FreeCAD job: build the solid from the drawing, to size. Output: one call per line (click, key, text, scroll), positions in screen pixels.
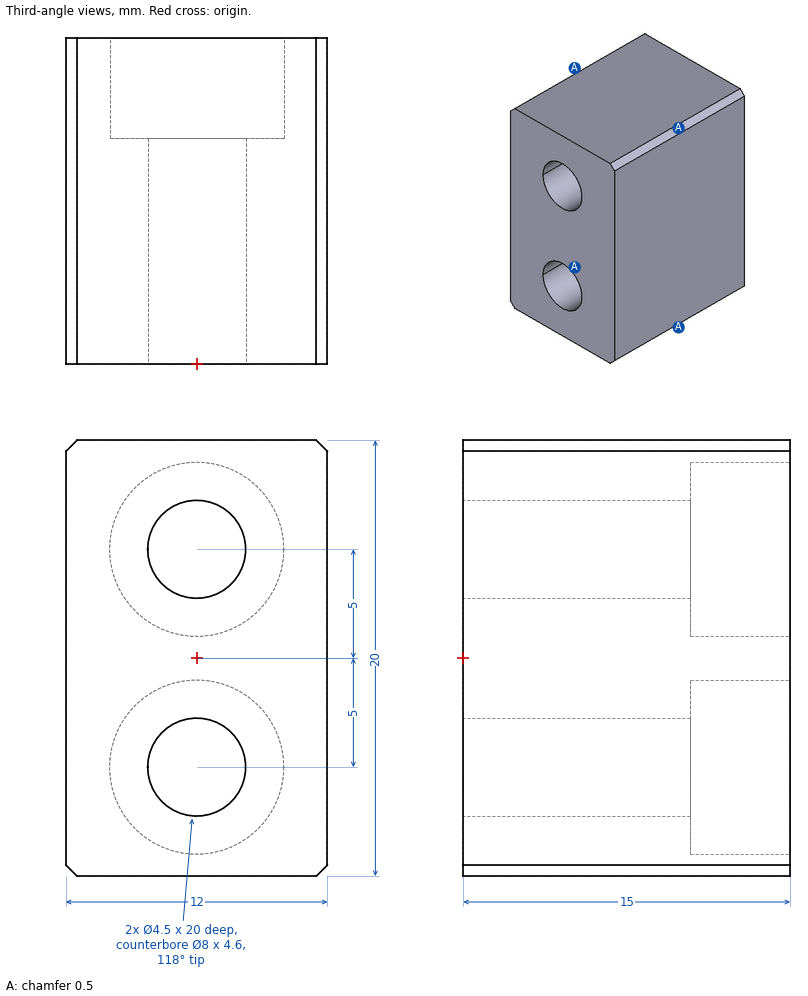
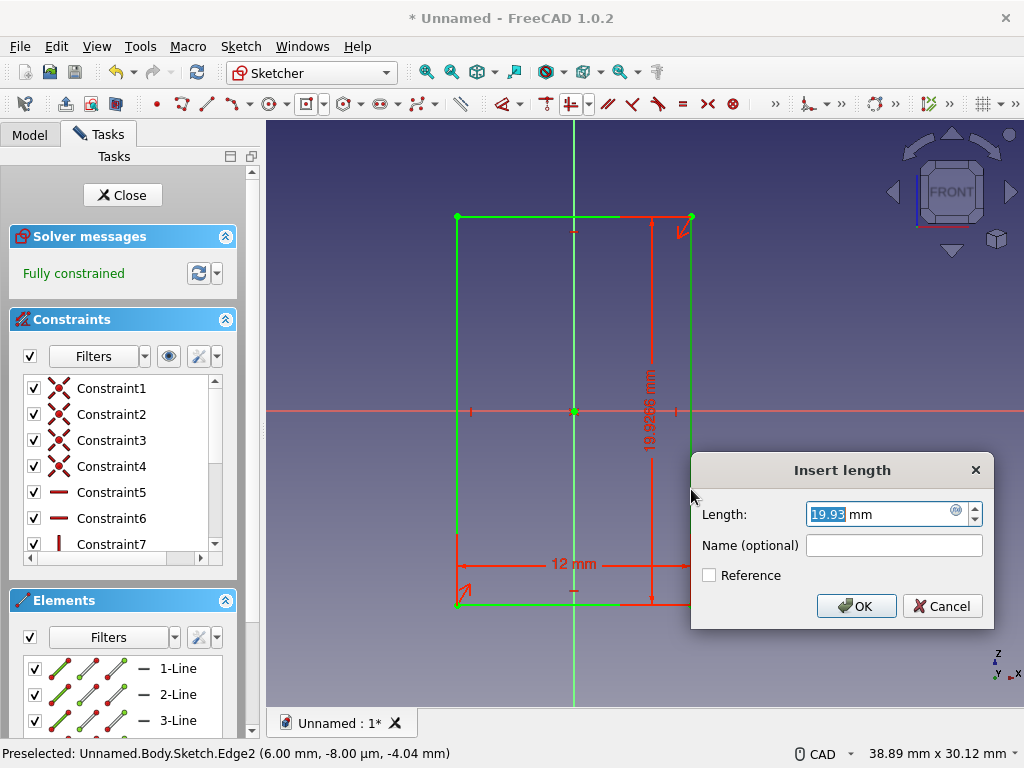
text(20)
key(Return)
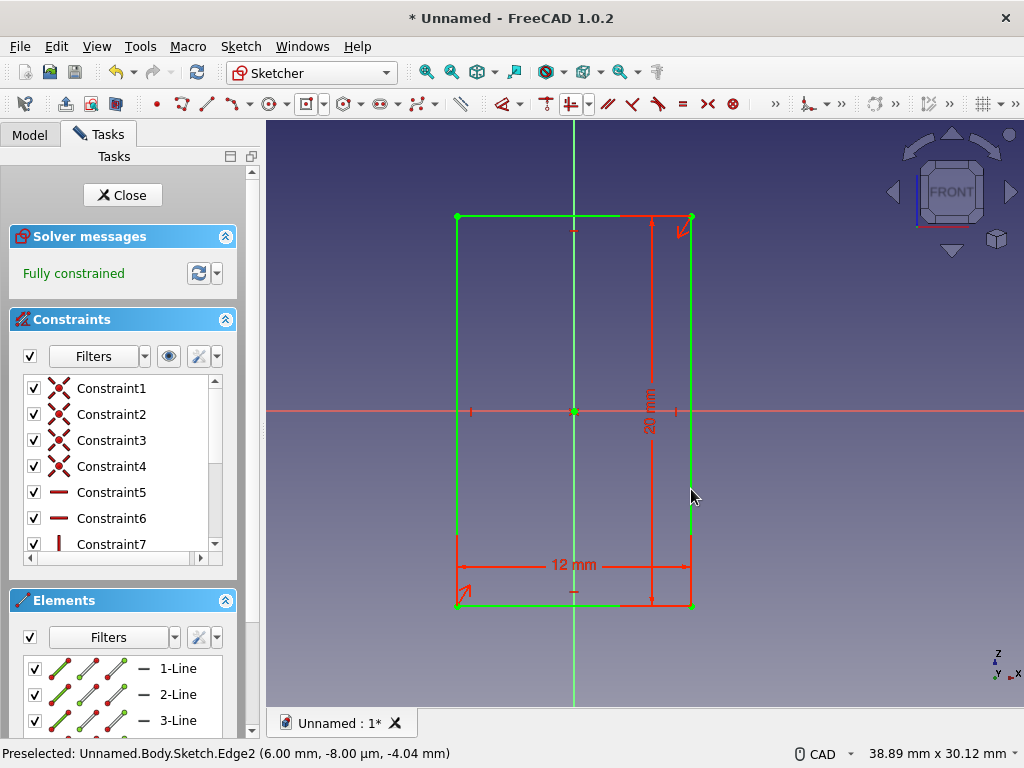
click(123, 195)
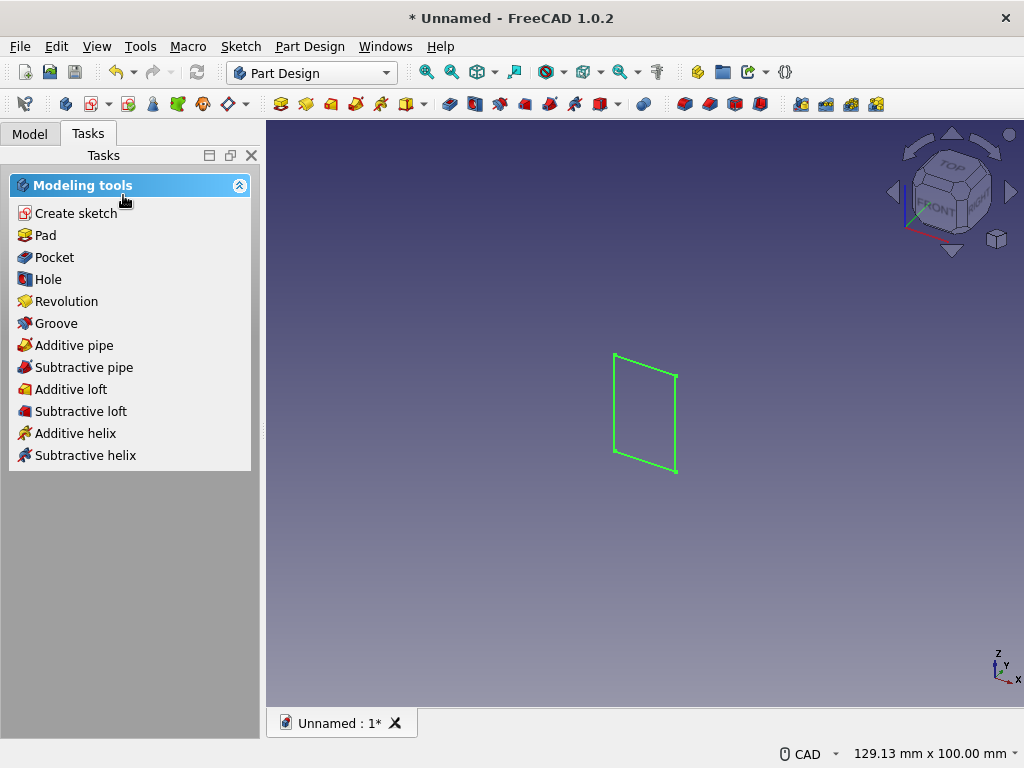
click(281, 104)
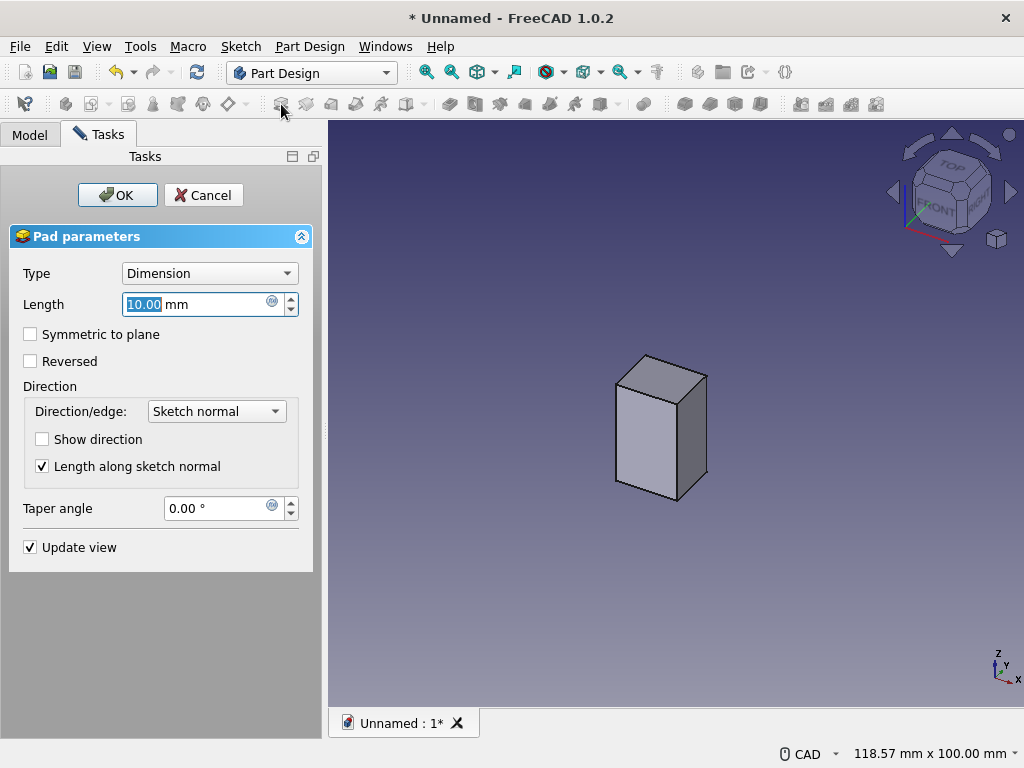
text(15)
key(Tab)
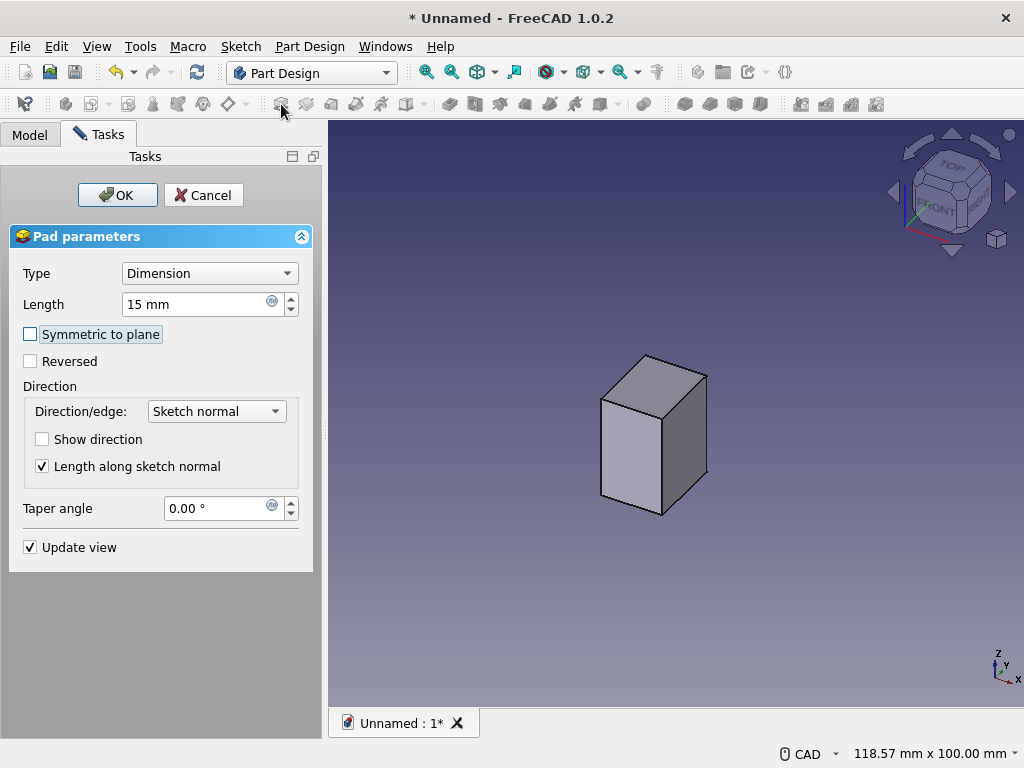
click(31, 361)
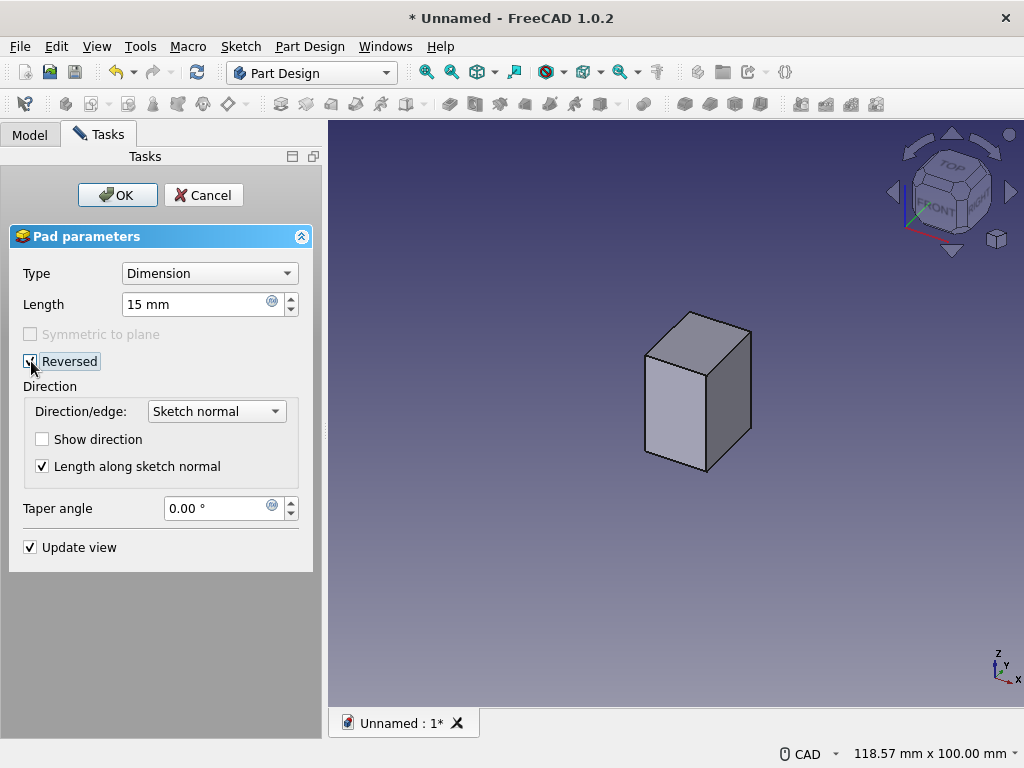
click(118, 195)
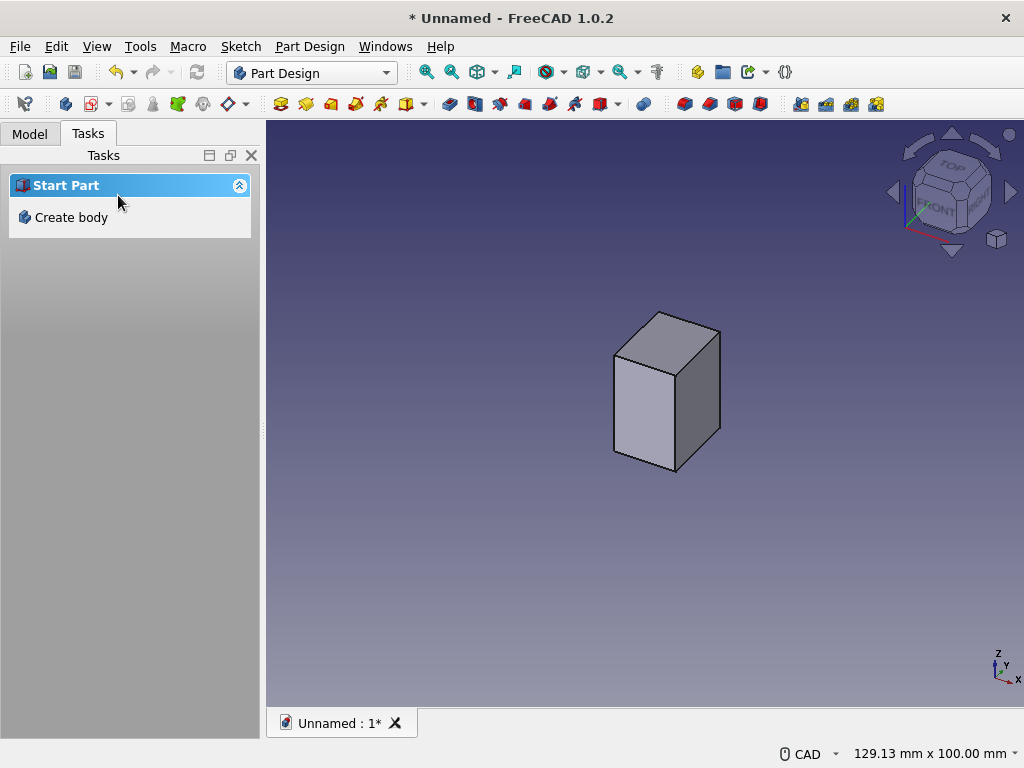
click(427, 72)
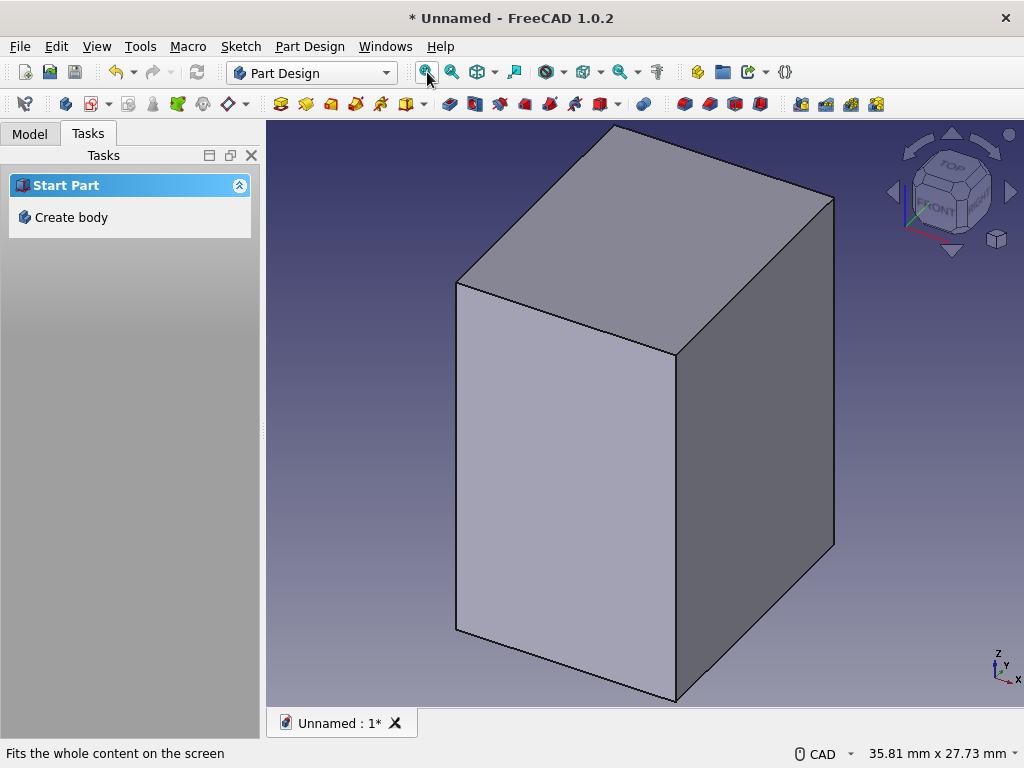
key(4)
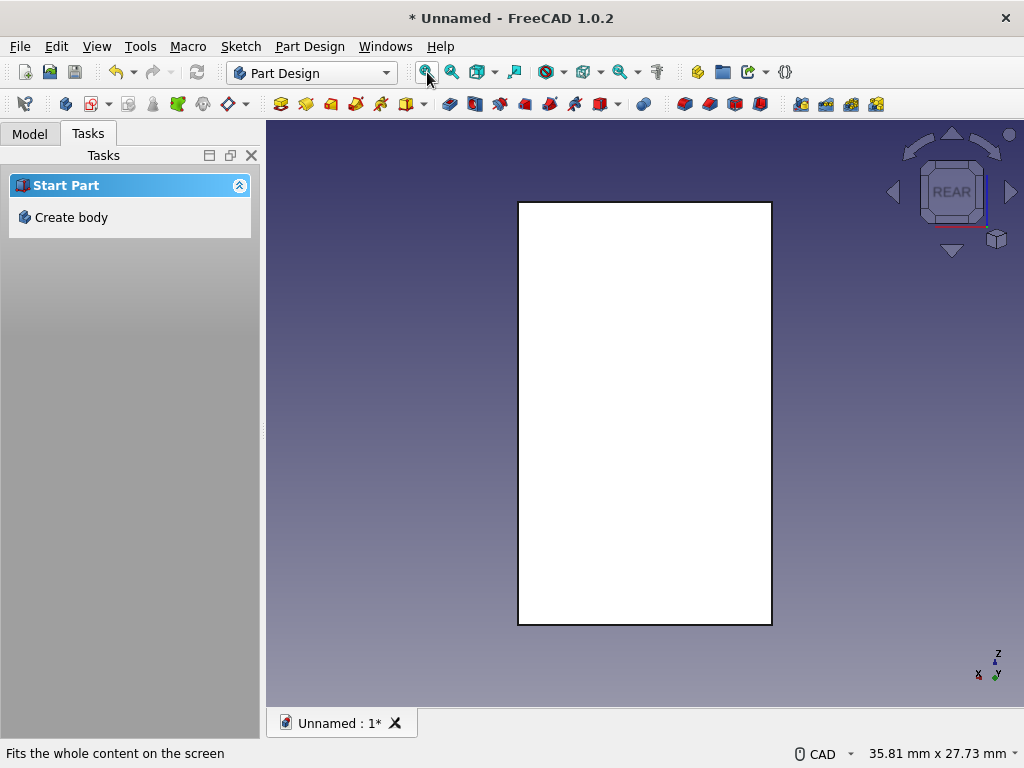
click(645, 352)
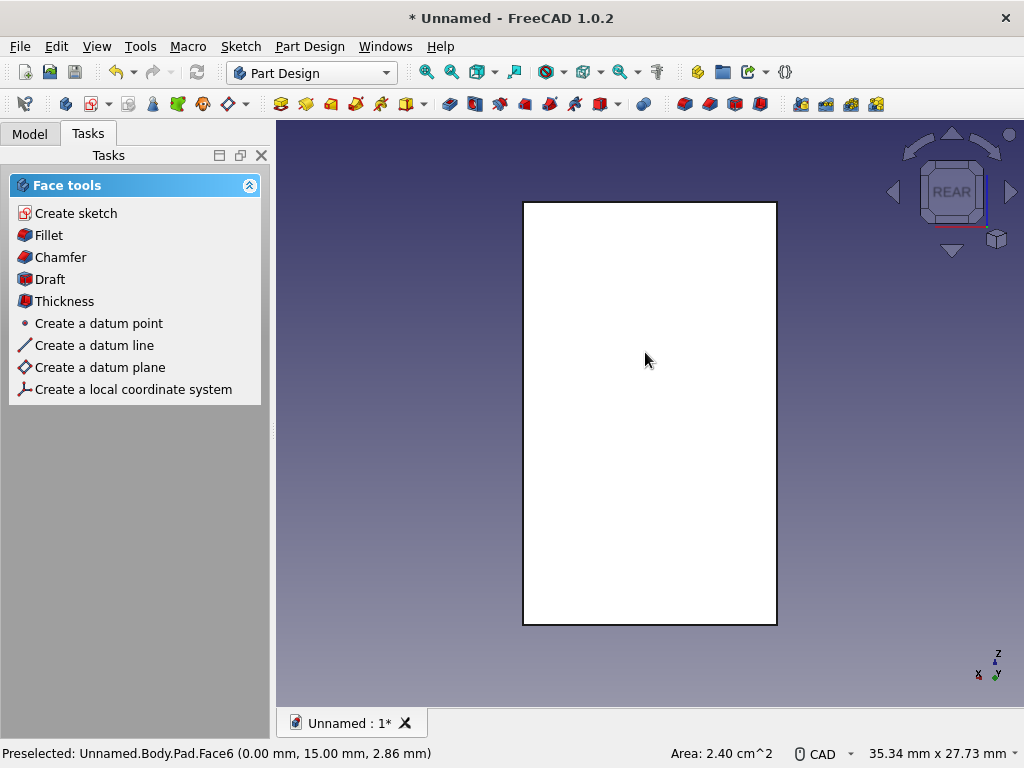
click(90, 104)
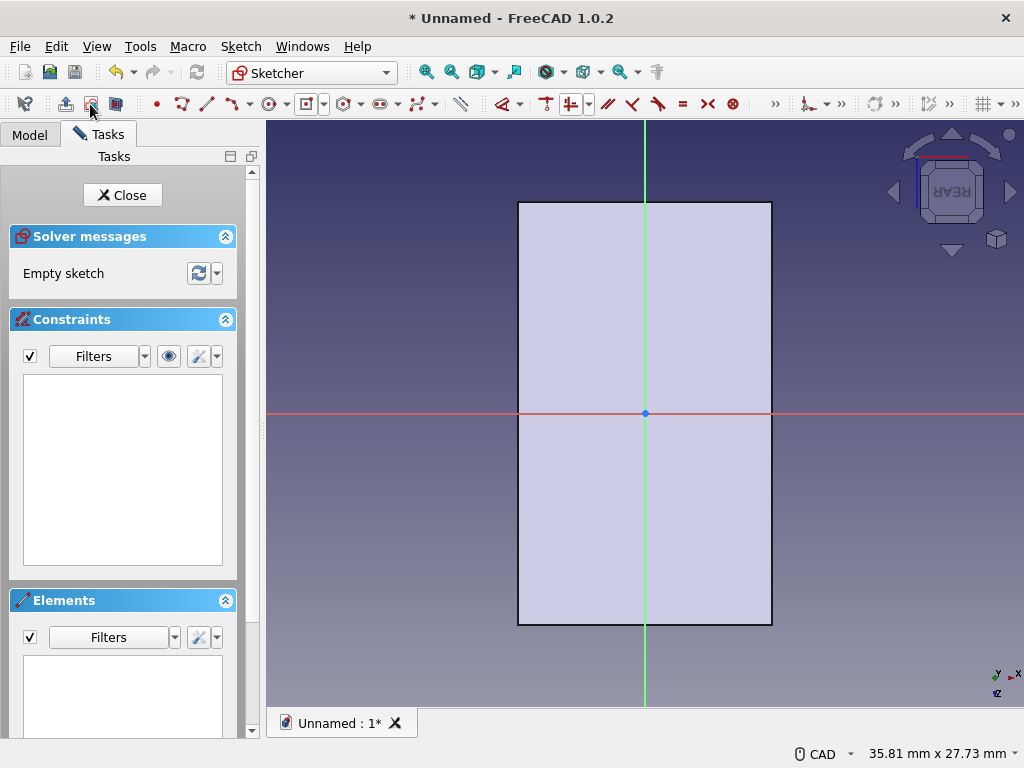
key(g)
key(c)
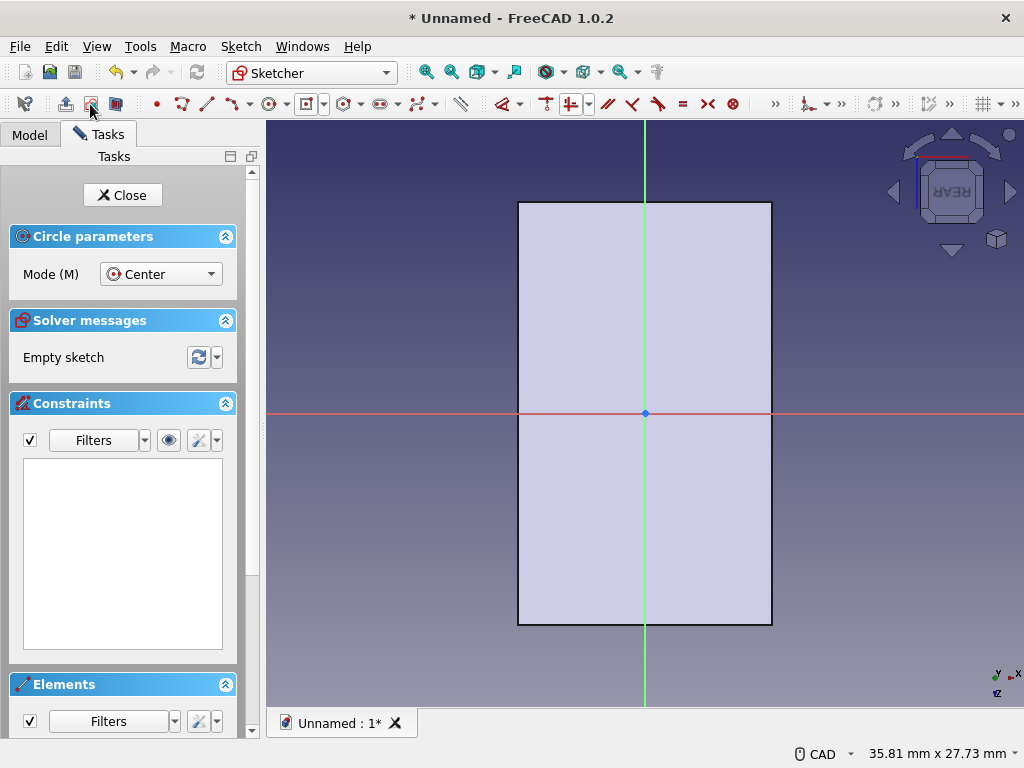
click(645, 308)
click(679, 274)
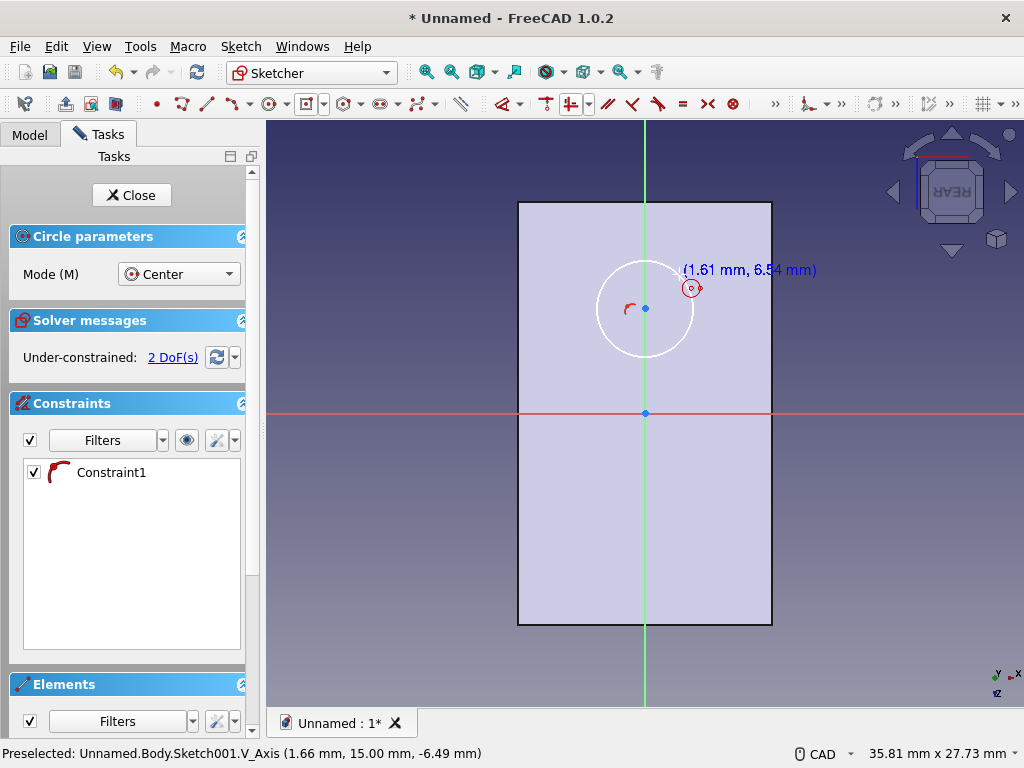
click(645, 519)
click(679, 486)
key(Escape)